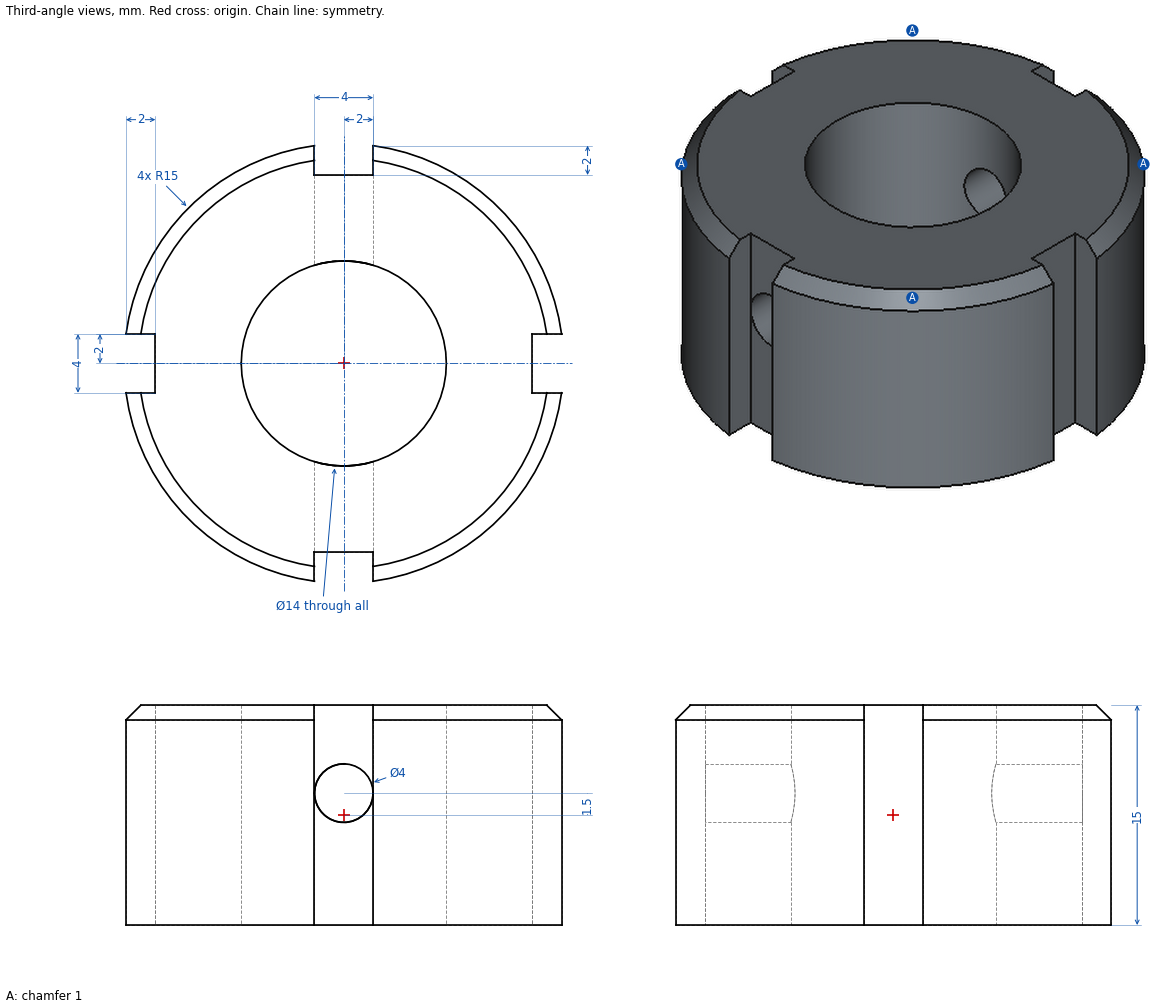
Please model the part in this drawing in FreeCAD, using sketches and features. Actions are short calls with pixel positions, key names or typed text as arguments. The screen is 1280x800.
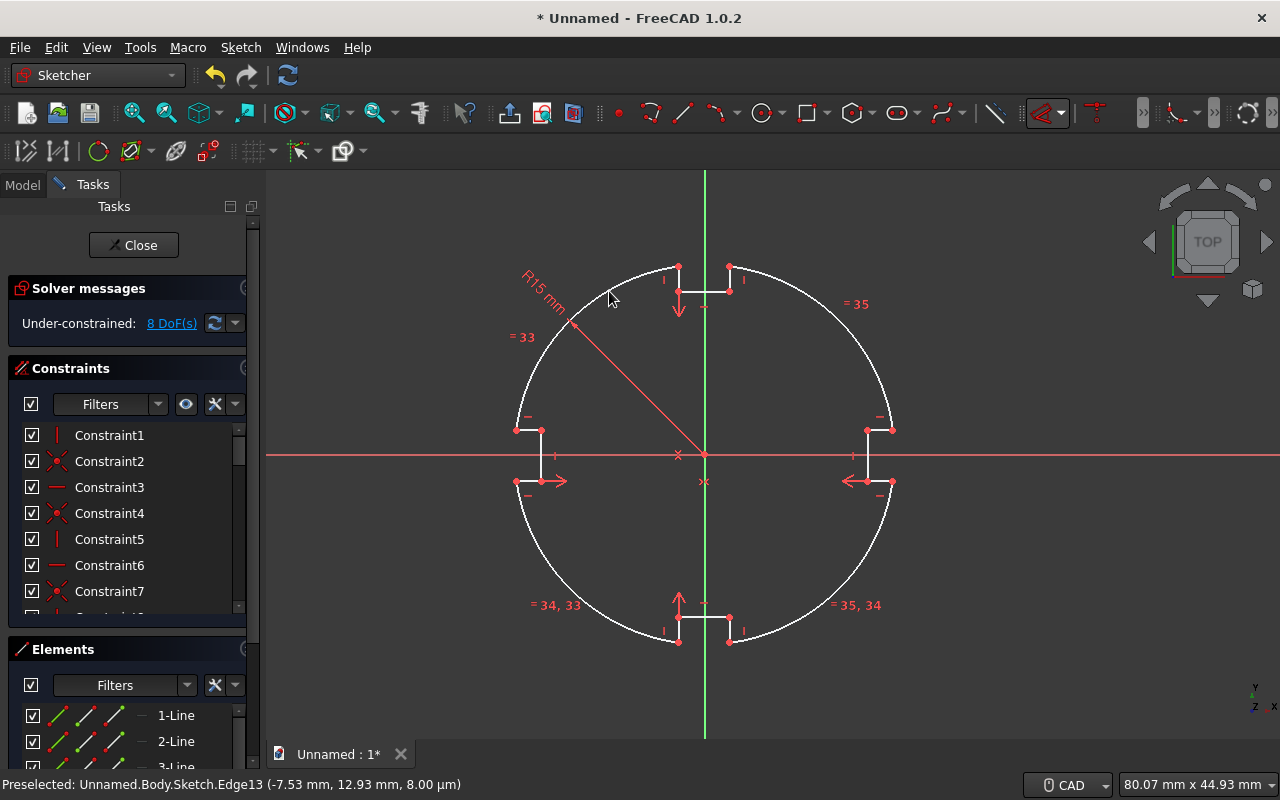
scroll(730, 277, up, 3)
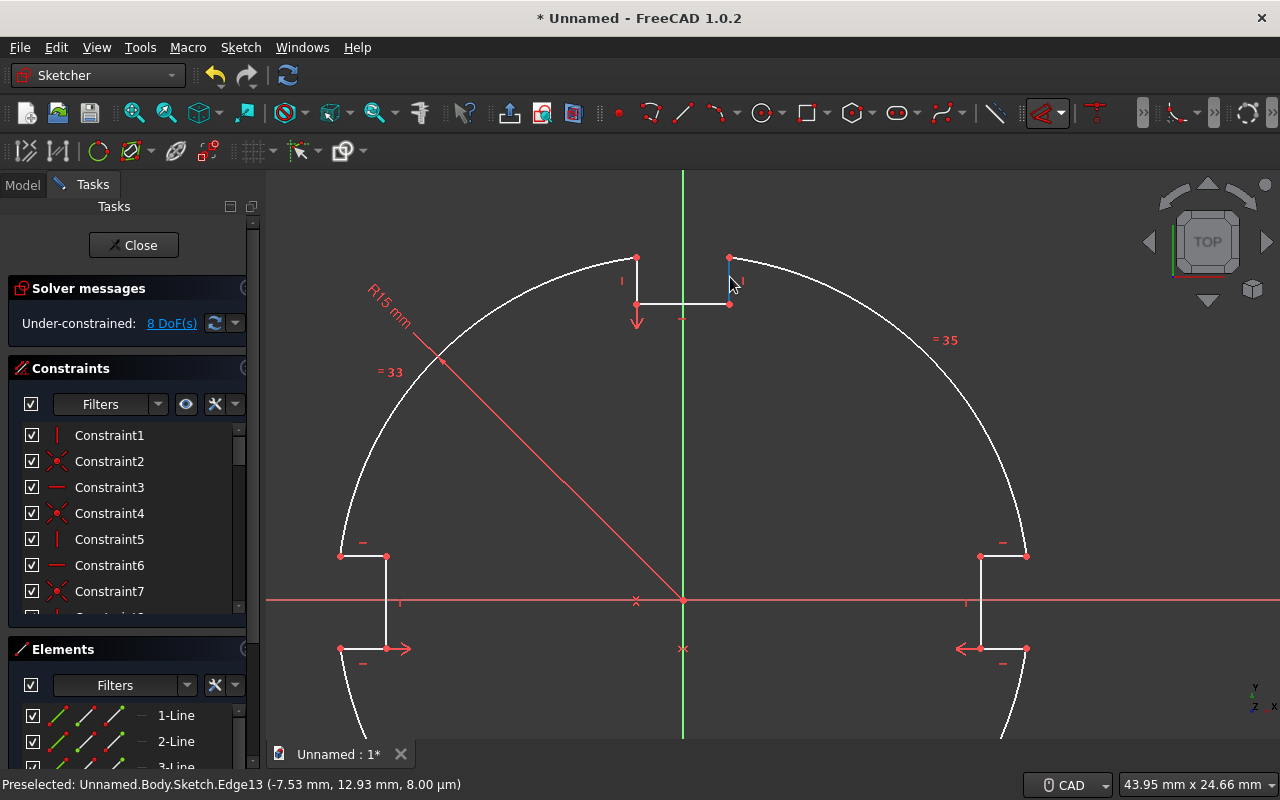
click(729, 276)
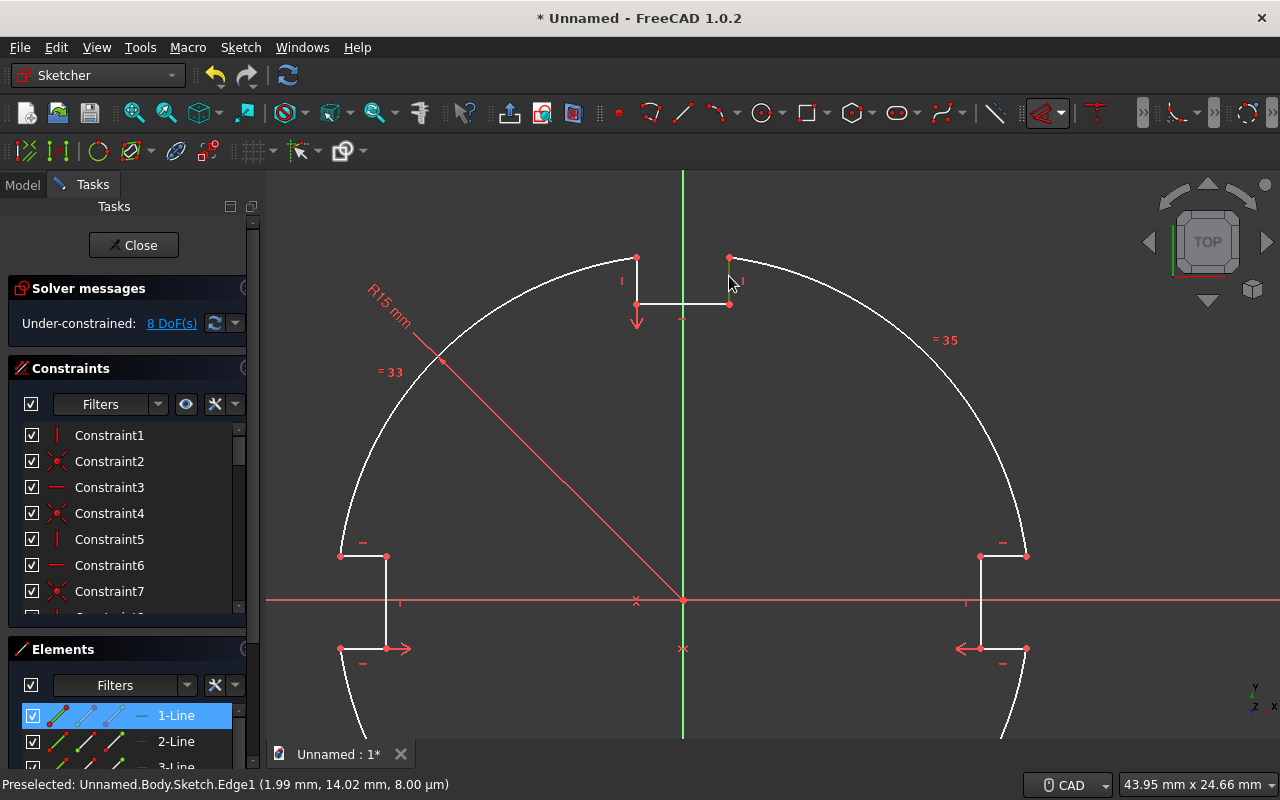
key(i)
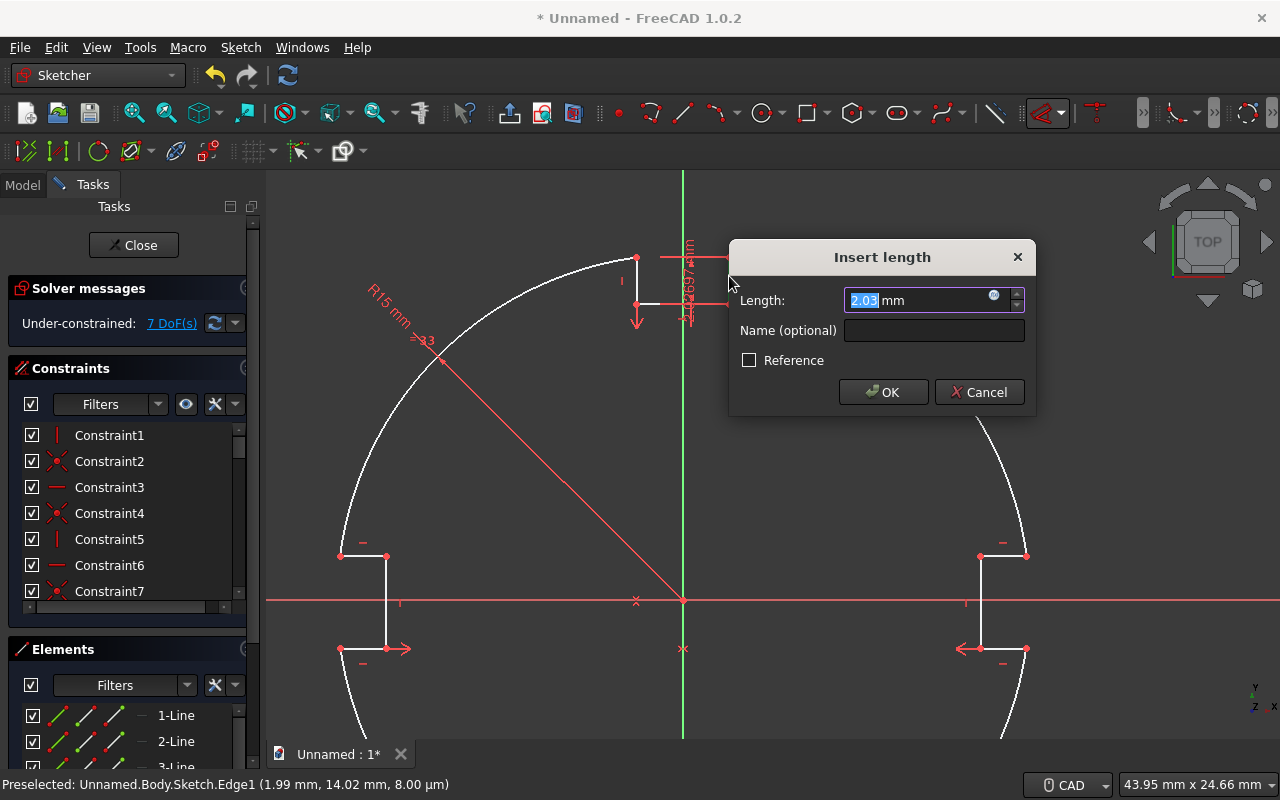
text(2)
key(Return)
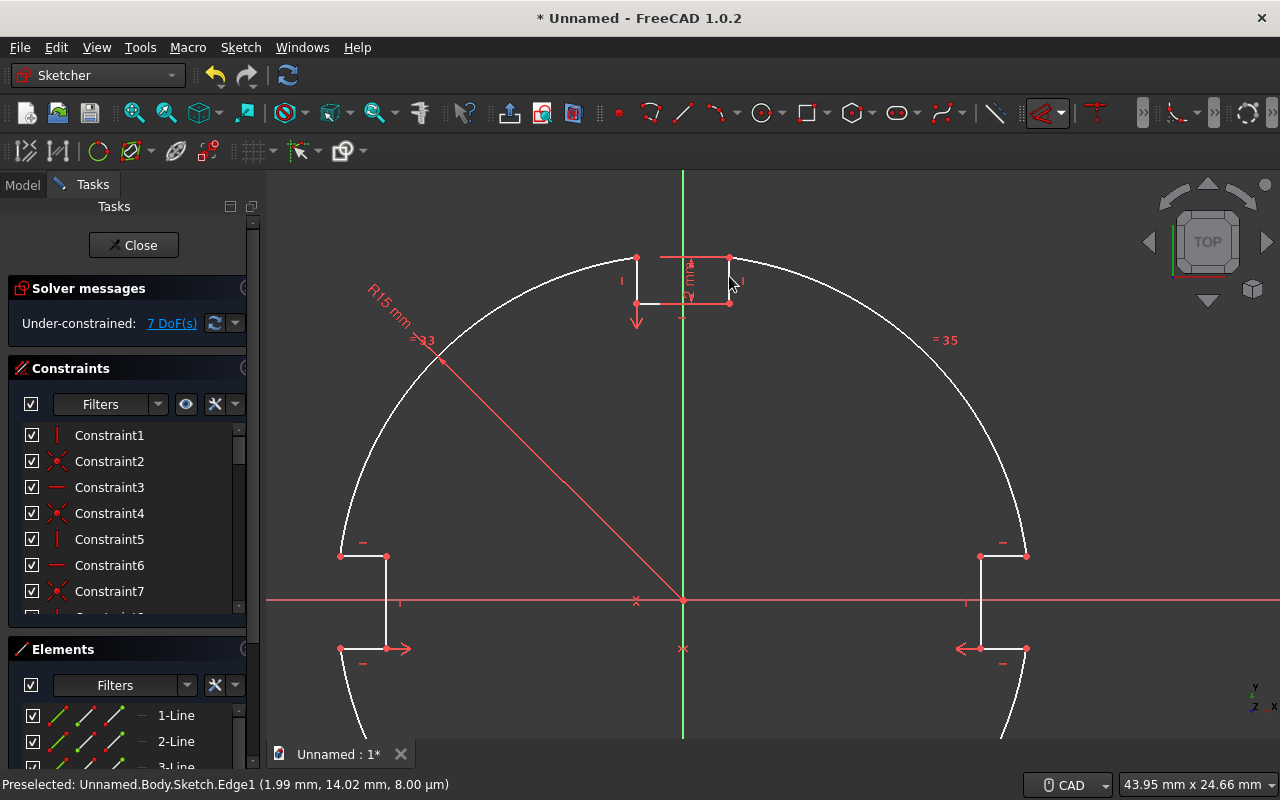
click(702, 304)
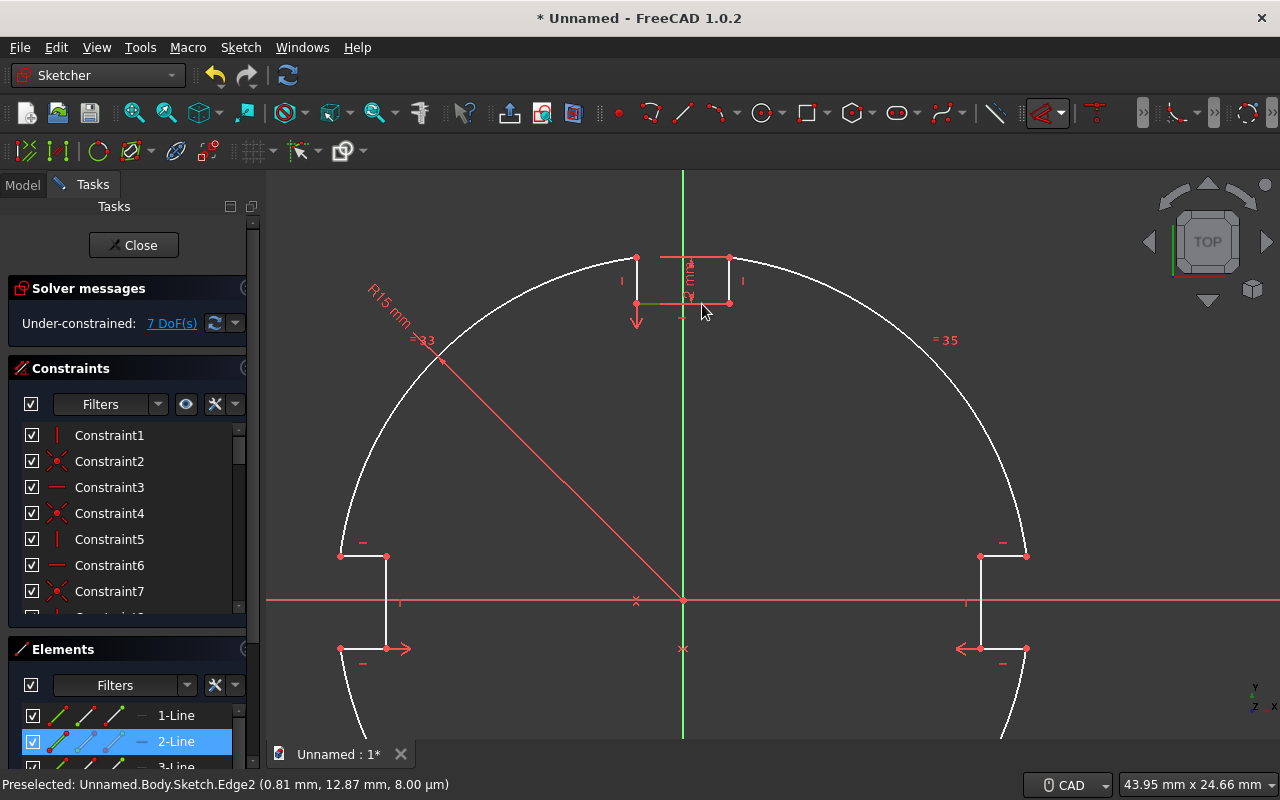
key(l)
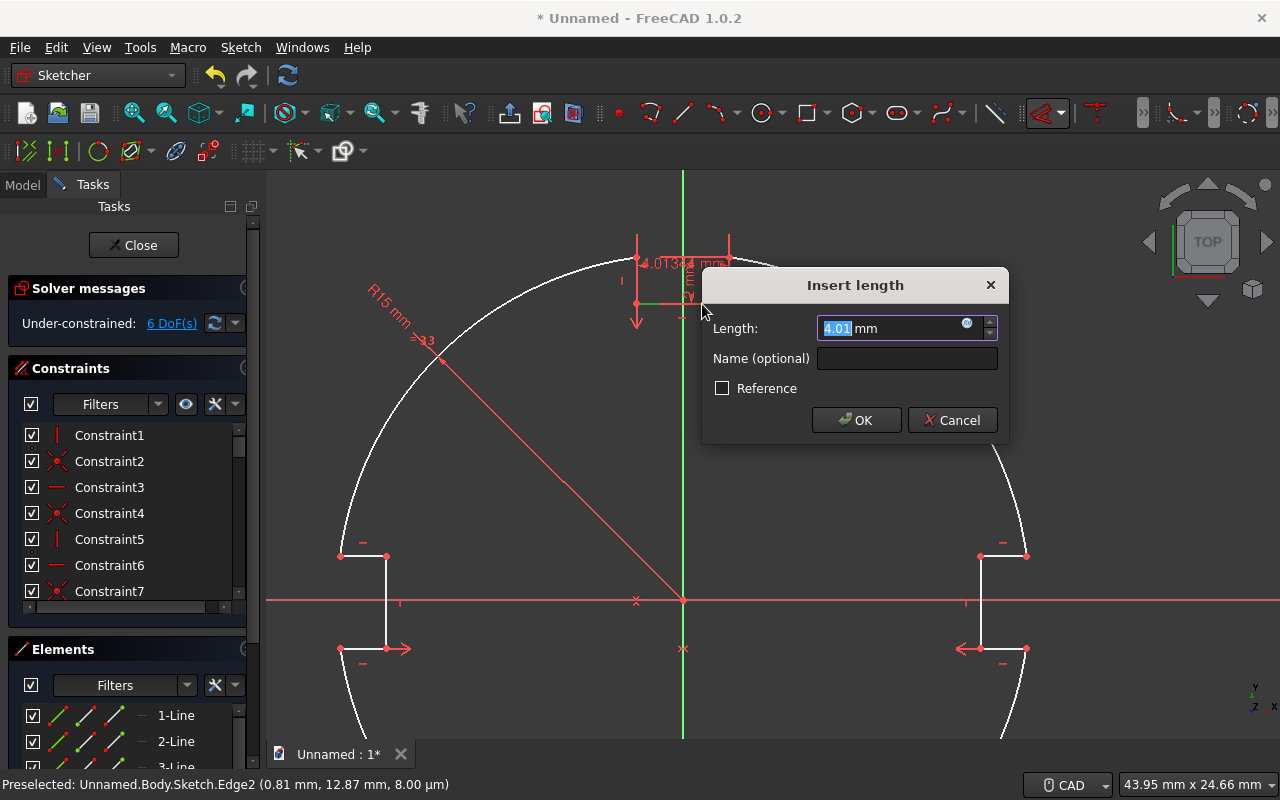
text(4)
key(Return)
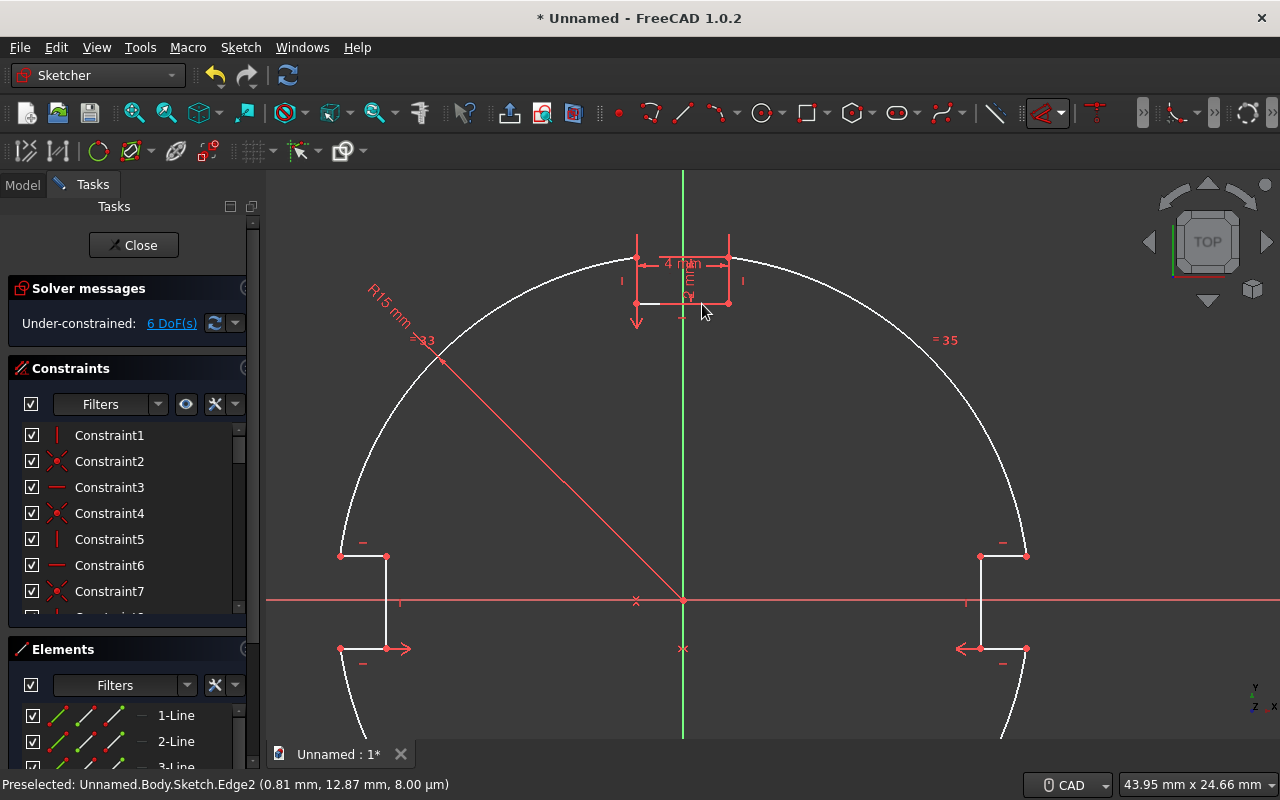
click(354, 556)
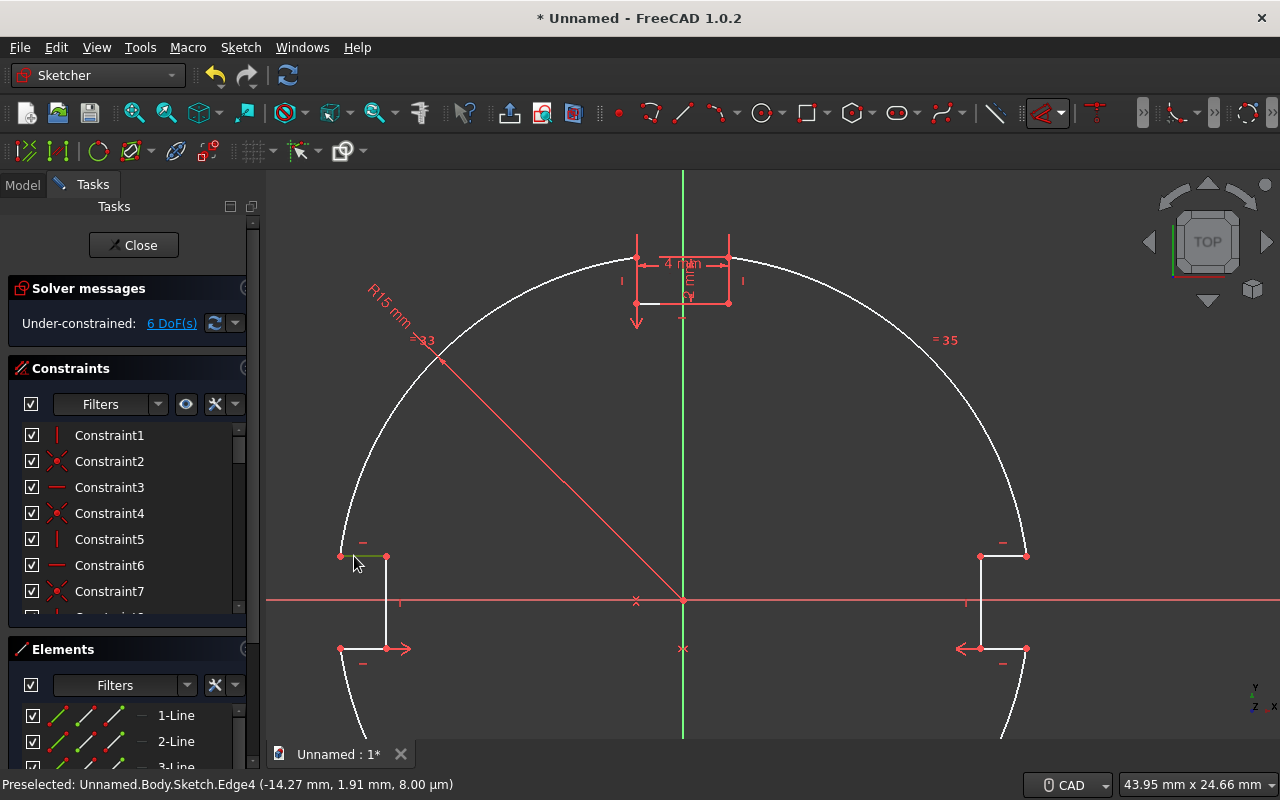
key(l)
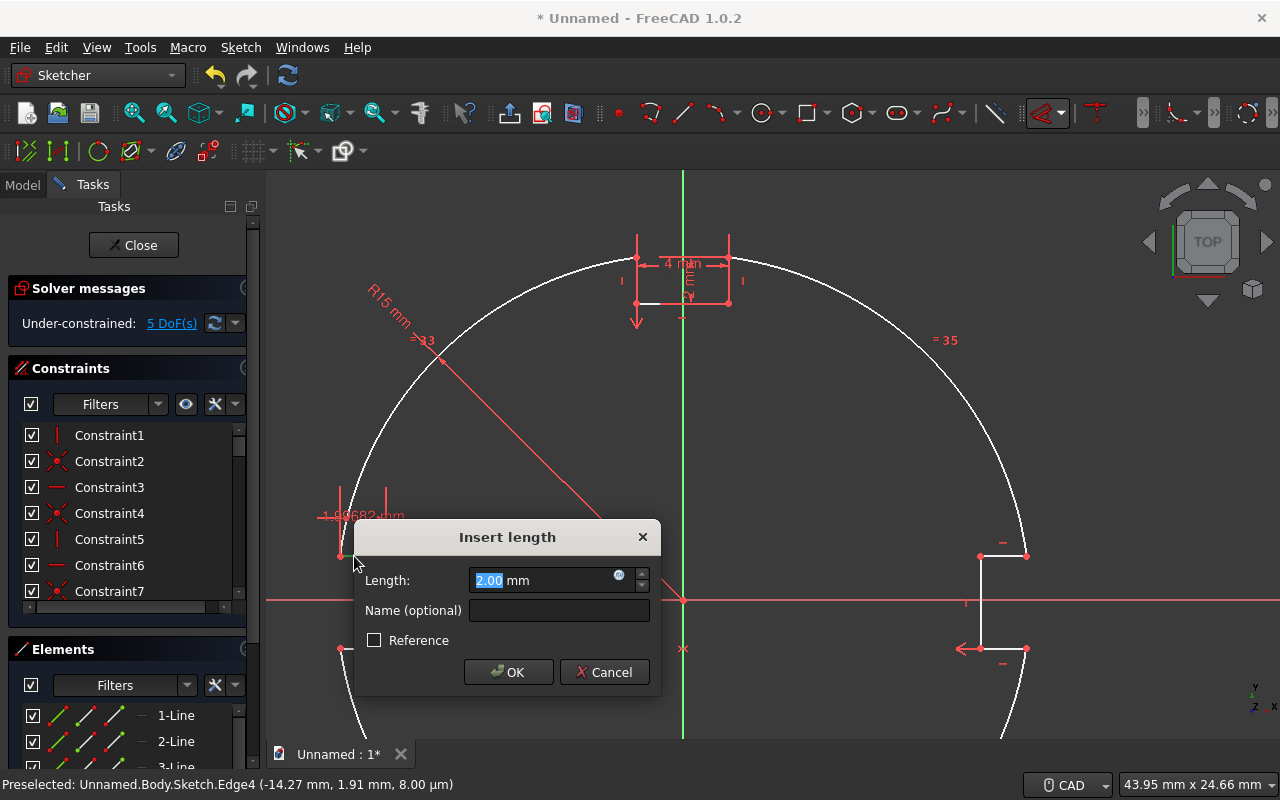
text(2)
key(Return)